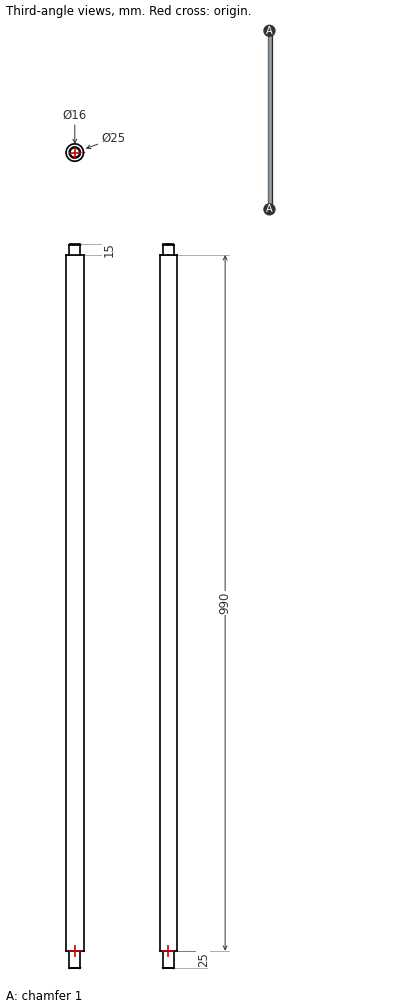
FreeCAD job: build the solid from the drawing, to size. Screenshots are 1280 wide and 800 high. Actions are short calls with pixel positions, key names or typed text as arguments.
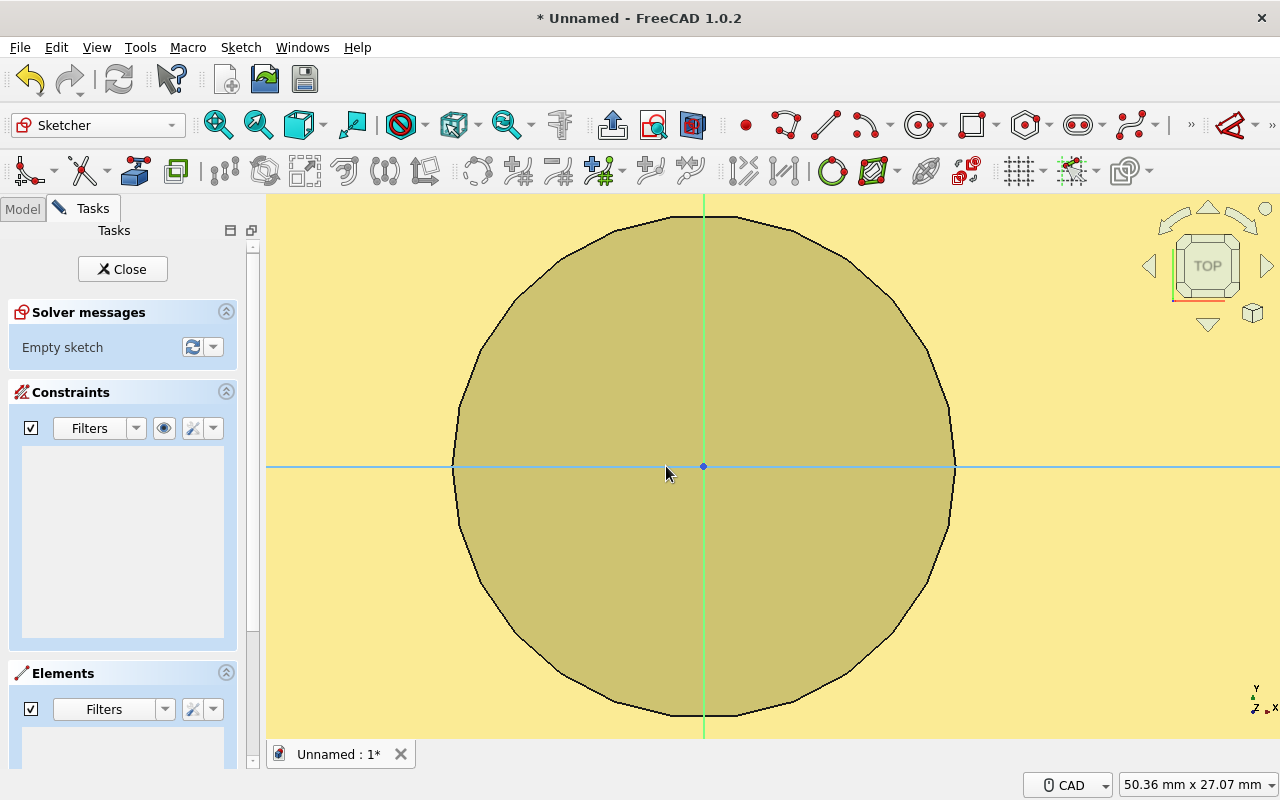
click(920, 126)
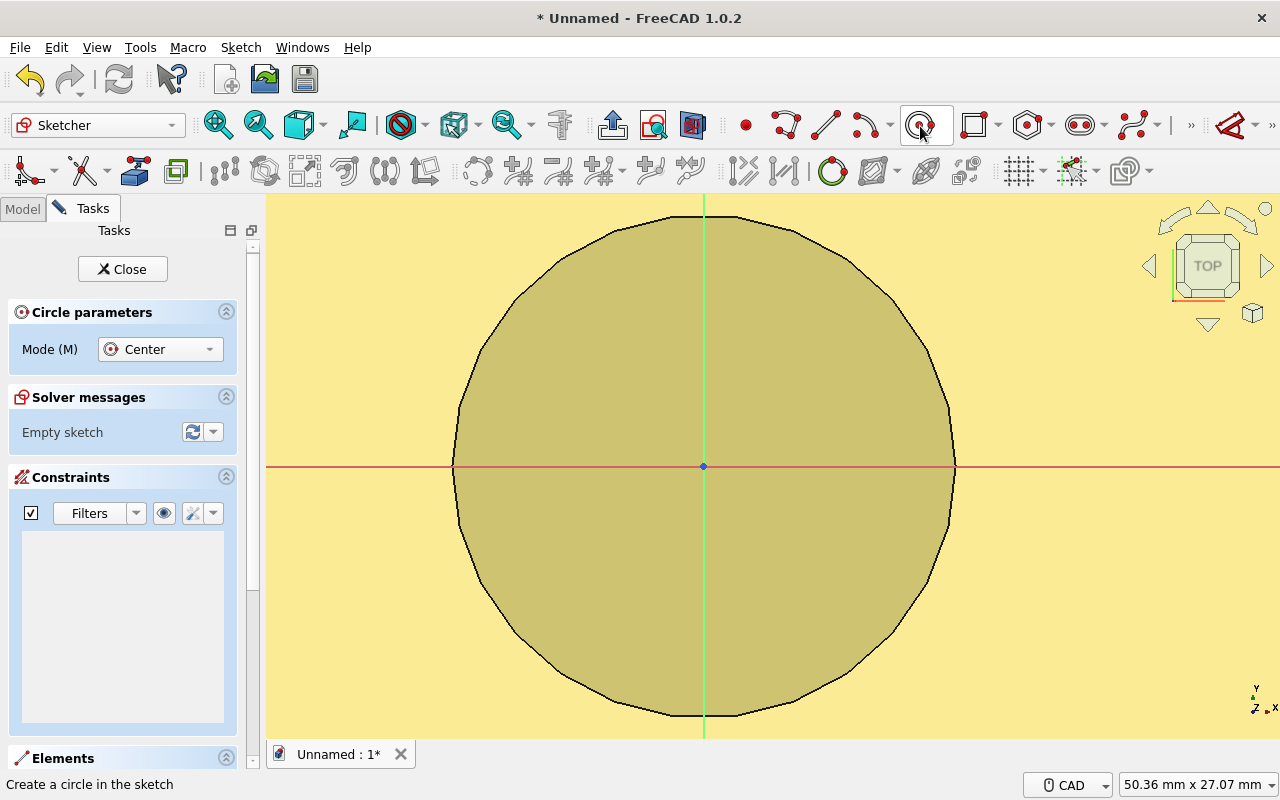
click(704, 466)
move(818, 353)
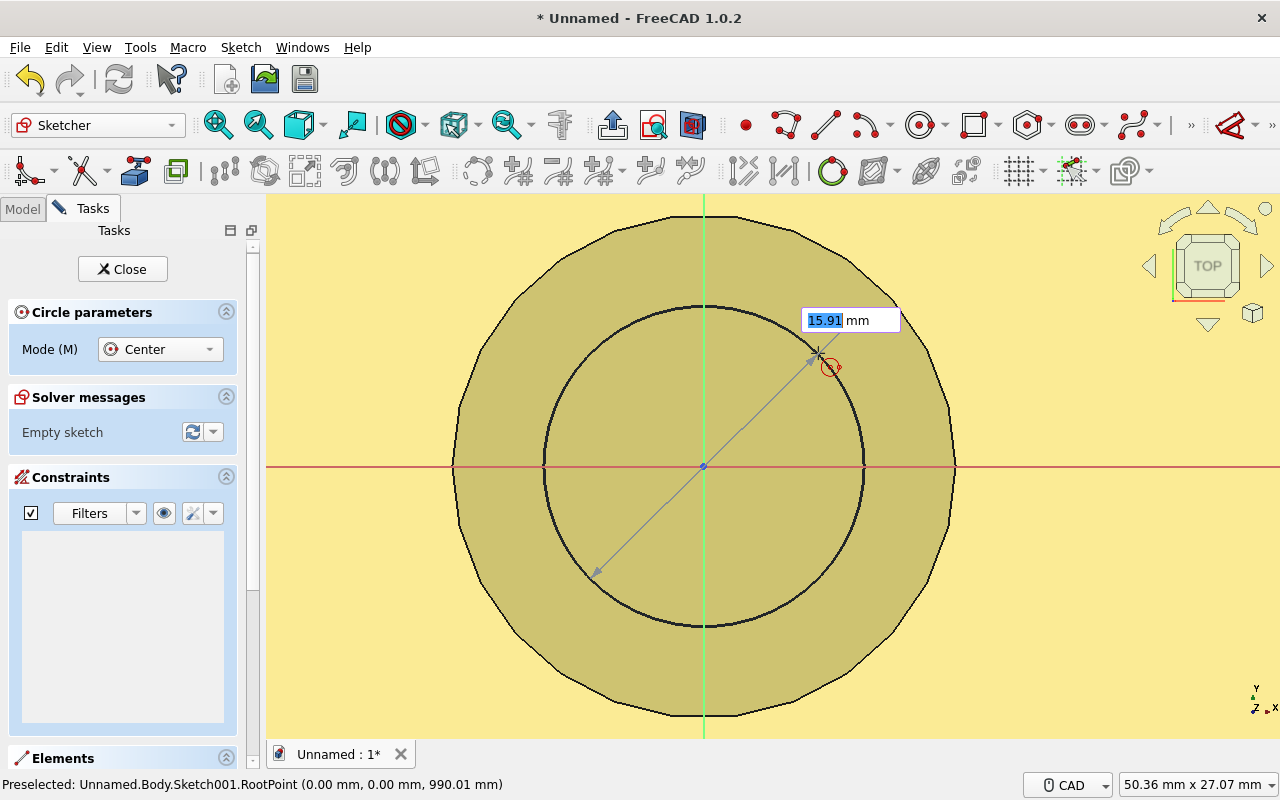
text(16)
key(Return)
key(Escape)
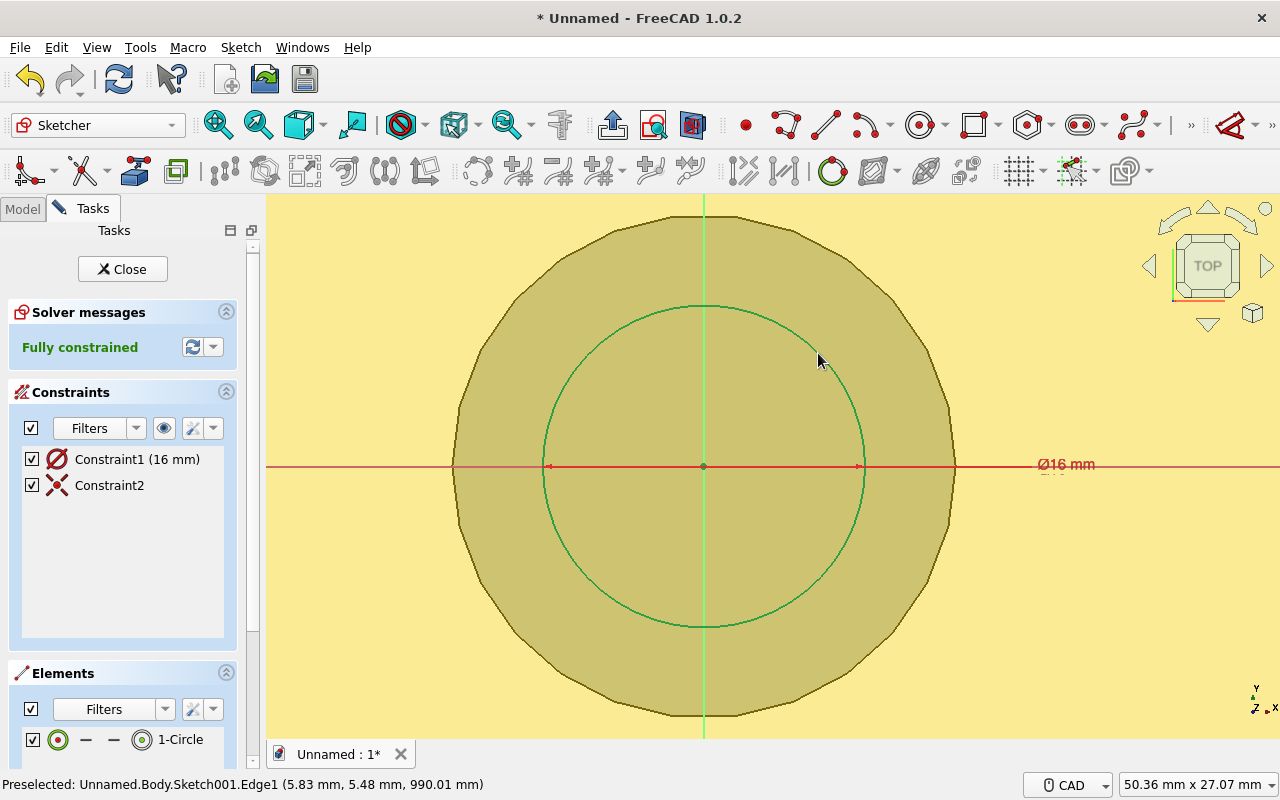
click(123, 269)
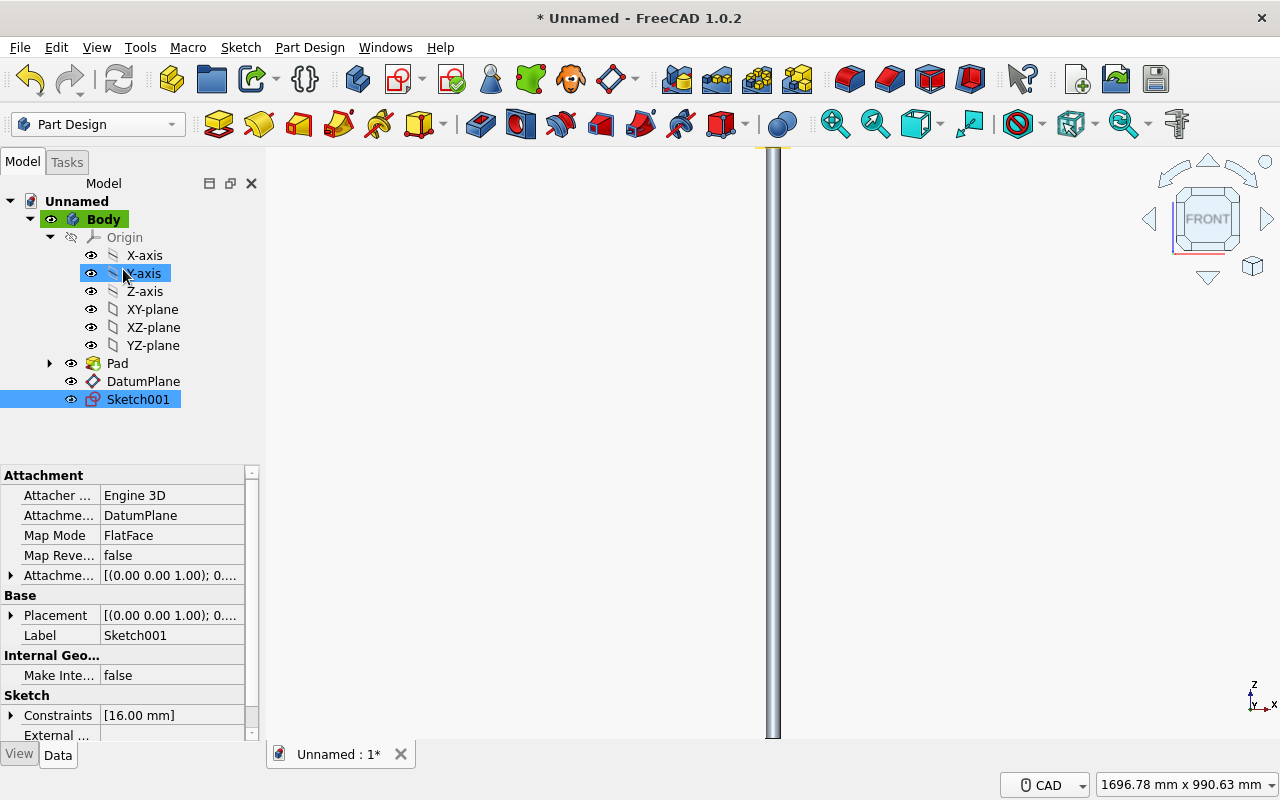
click(220, 124)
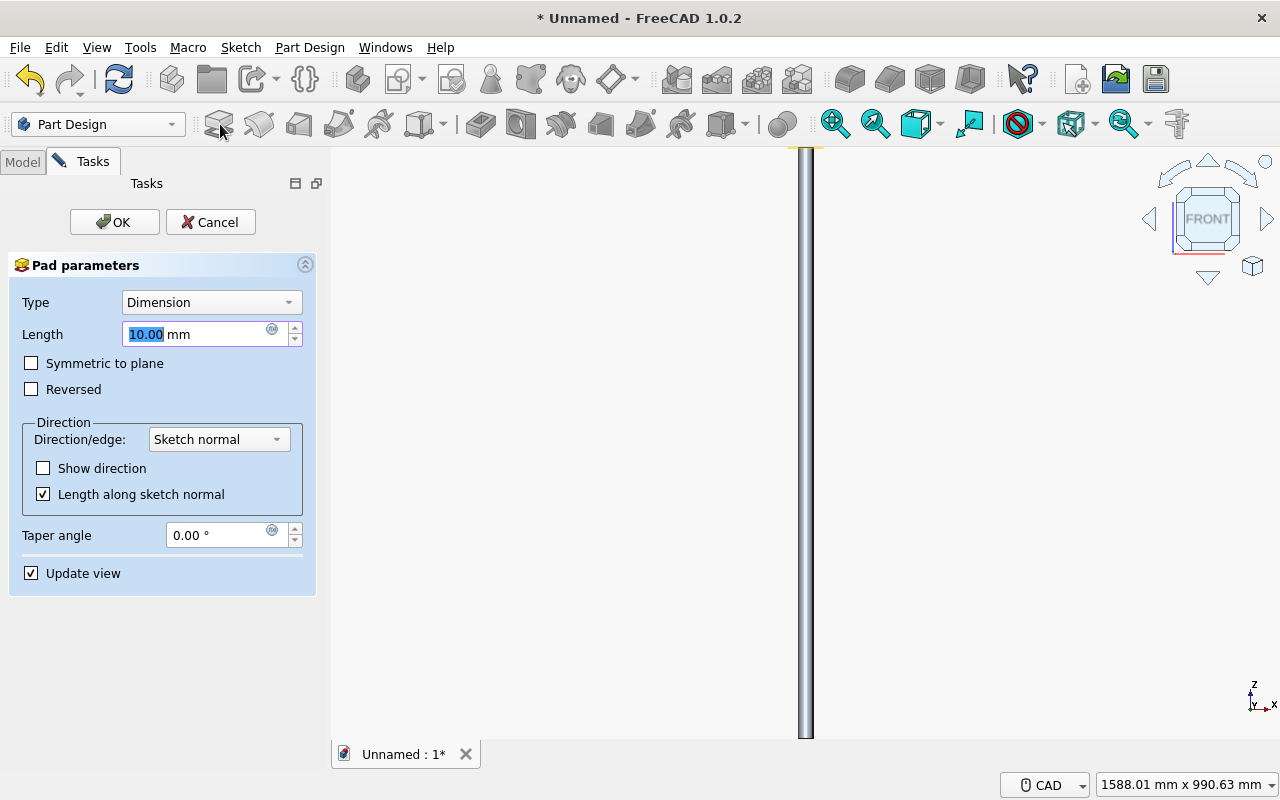
text(15)
key(Tab)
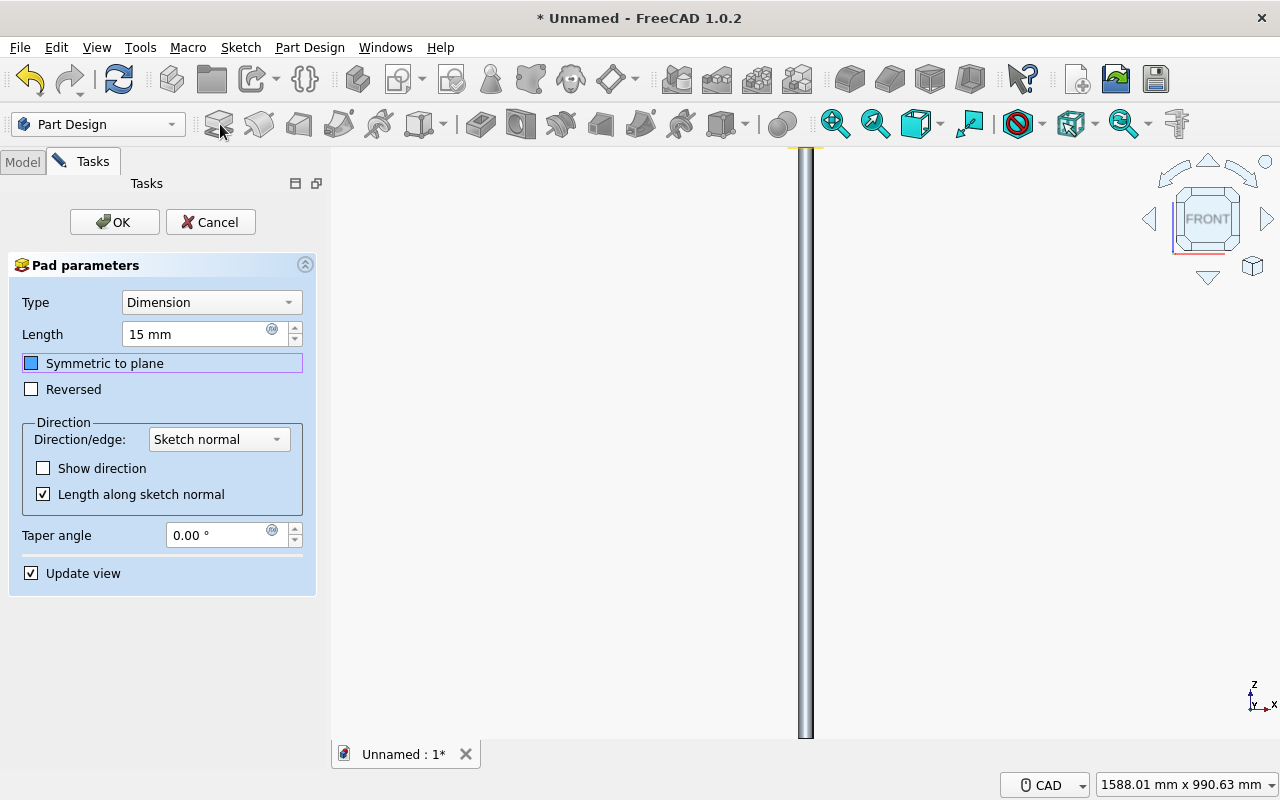
click(115, 222)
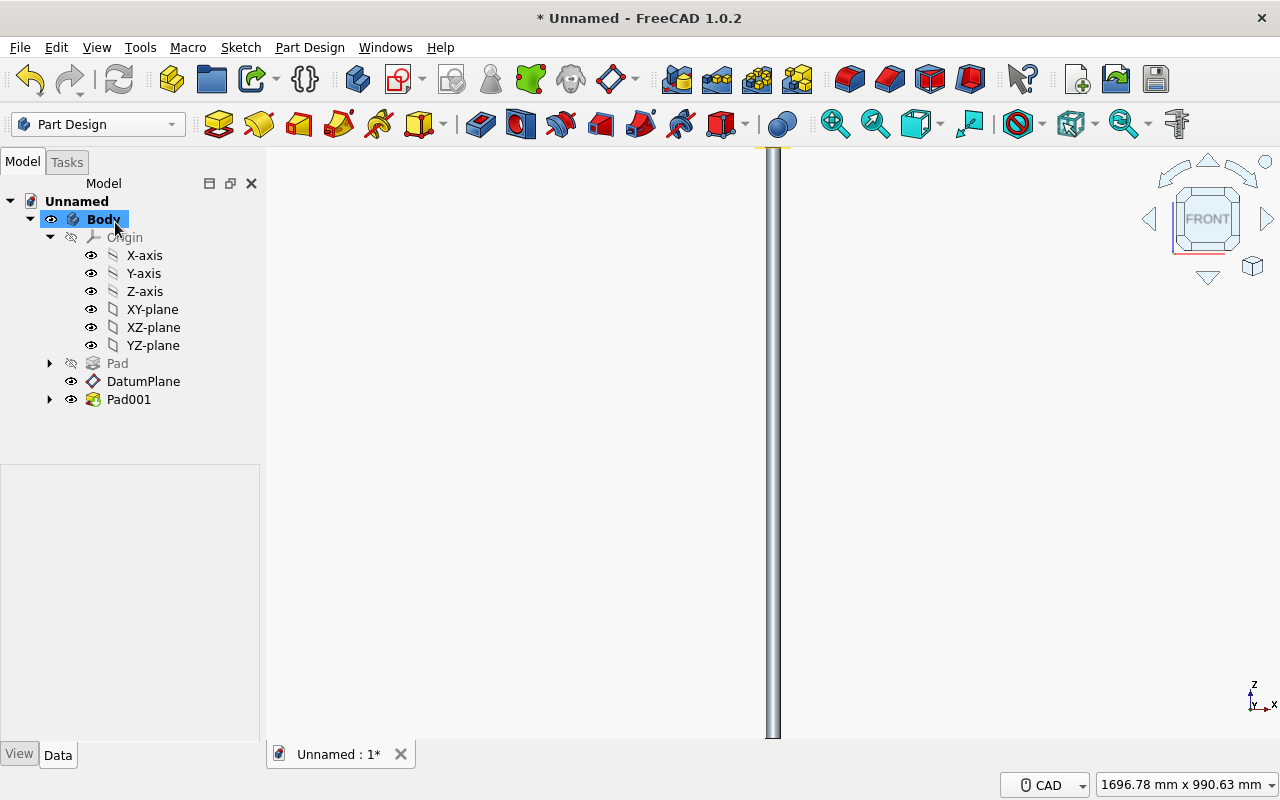
click(116, 381)
key(space)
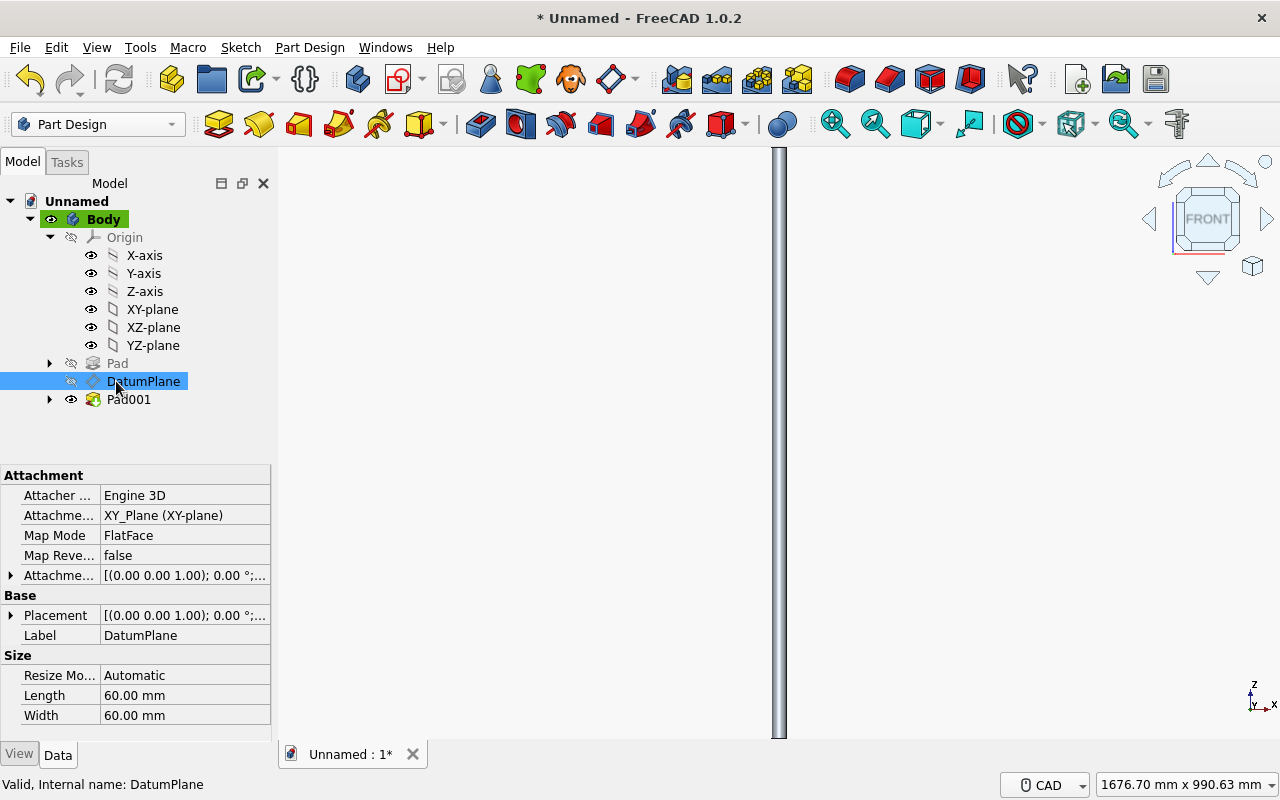
click(836, 124)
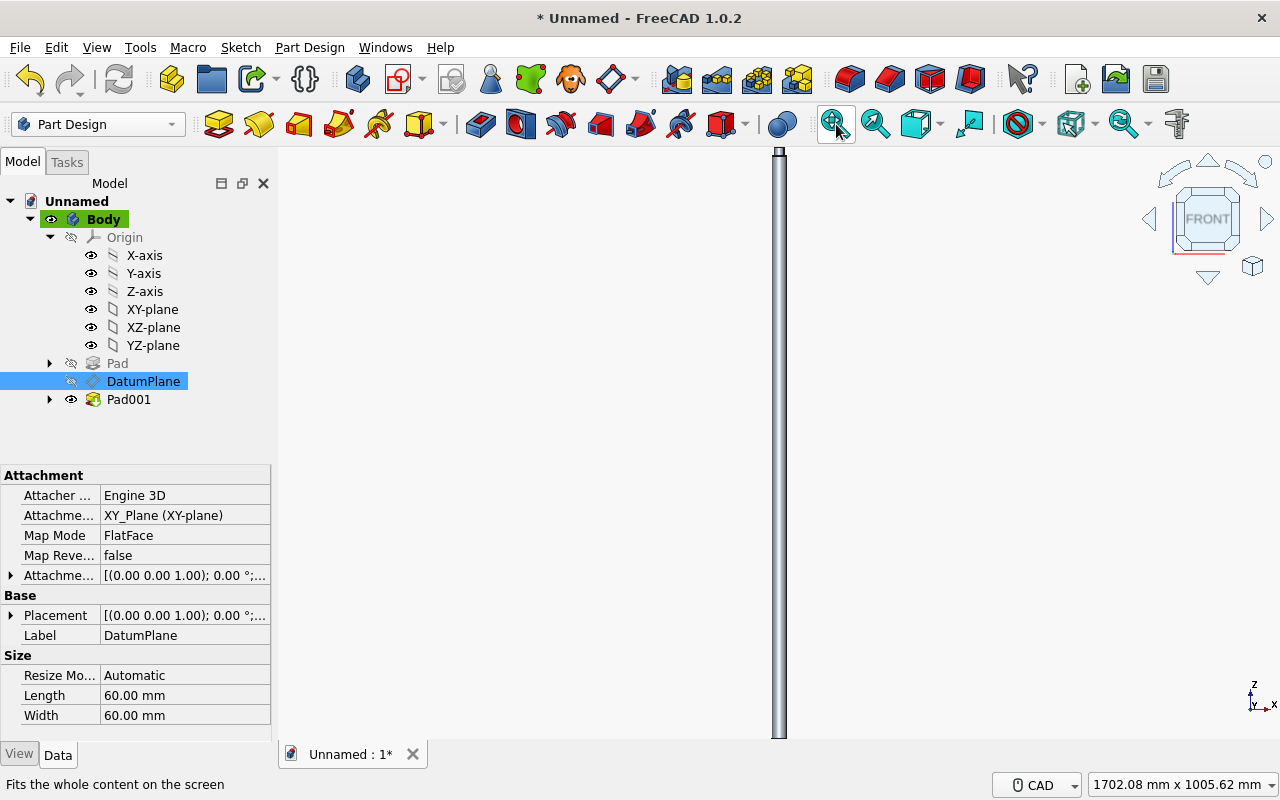
click(136, 309)